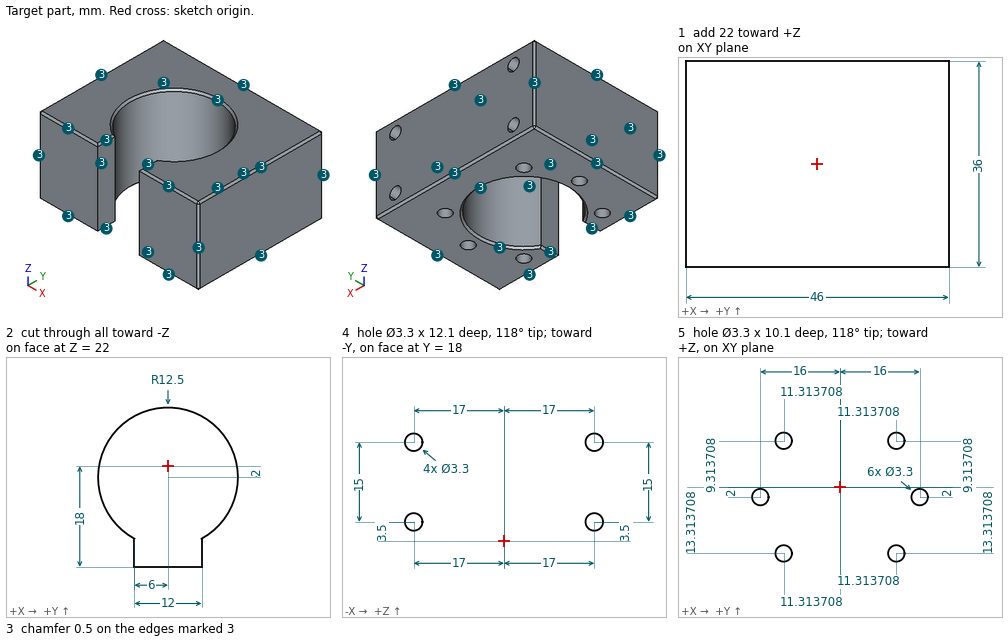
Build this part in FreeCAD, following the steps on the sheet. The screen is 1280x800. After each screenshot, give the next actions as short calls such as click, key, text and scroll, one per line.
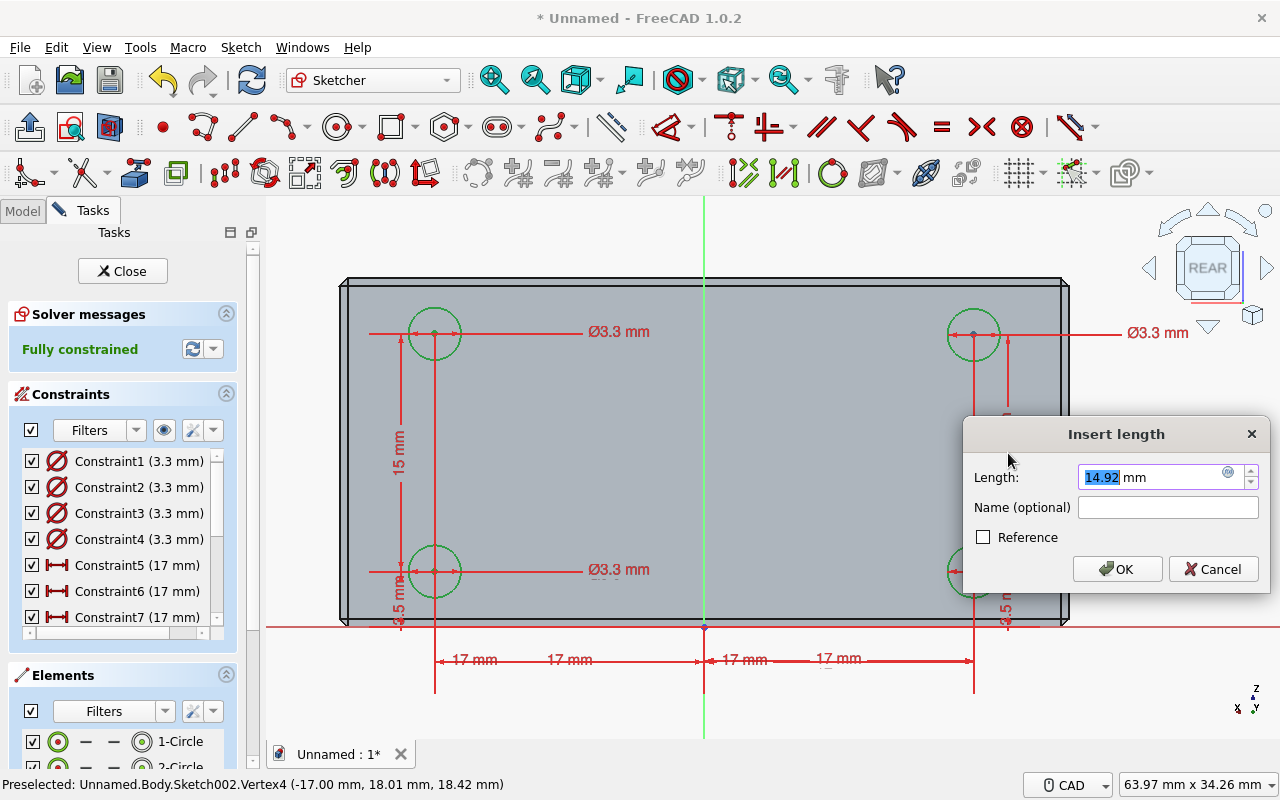
text(15)
key(Return)
key(Escape)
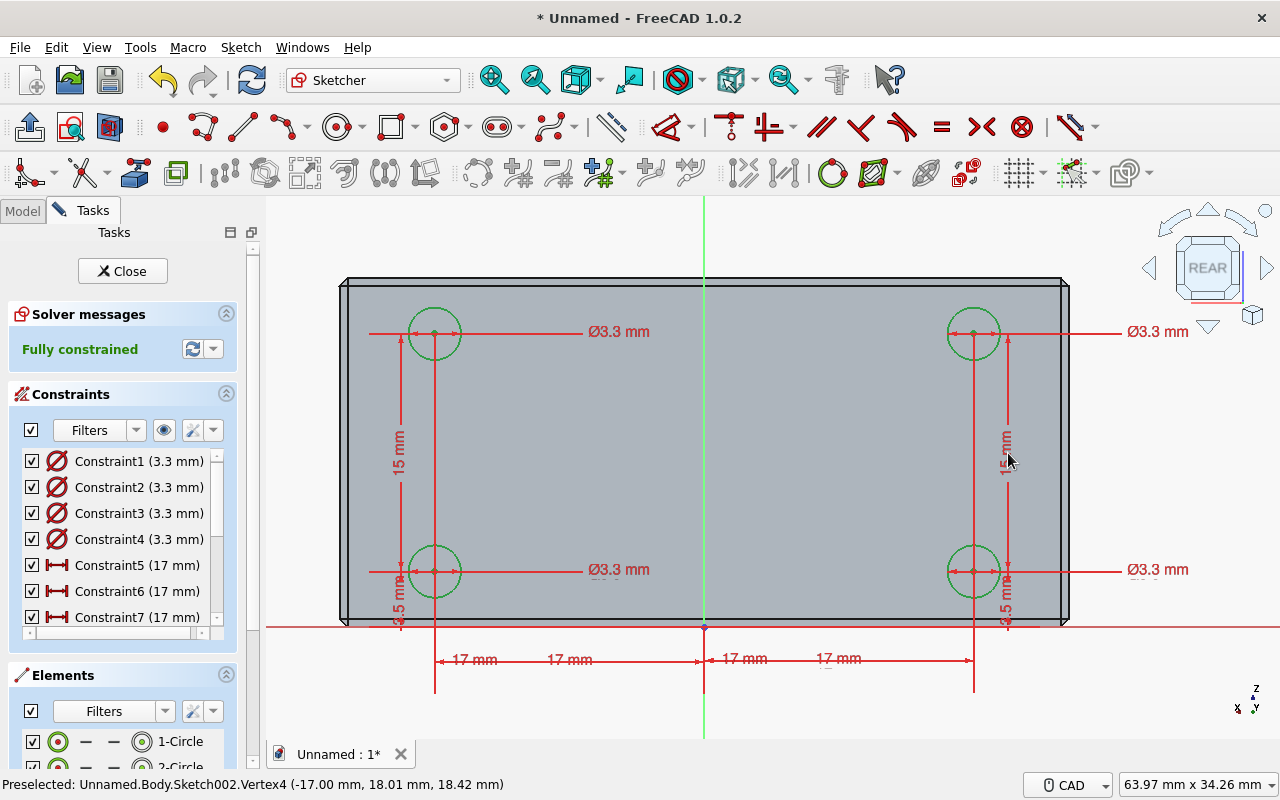
click(123, 271)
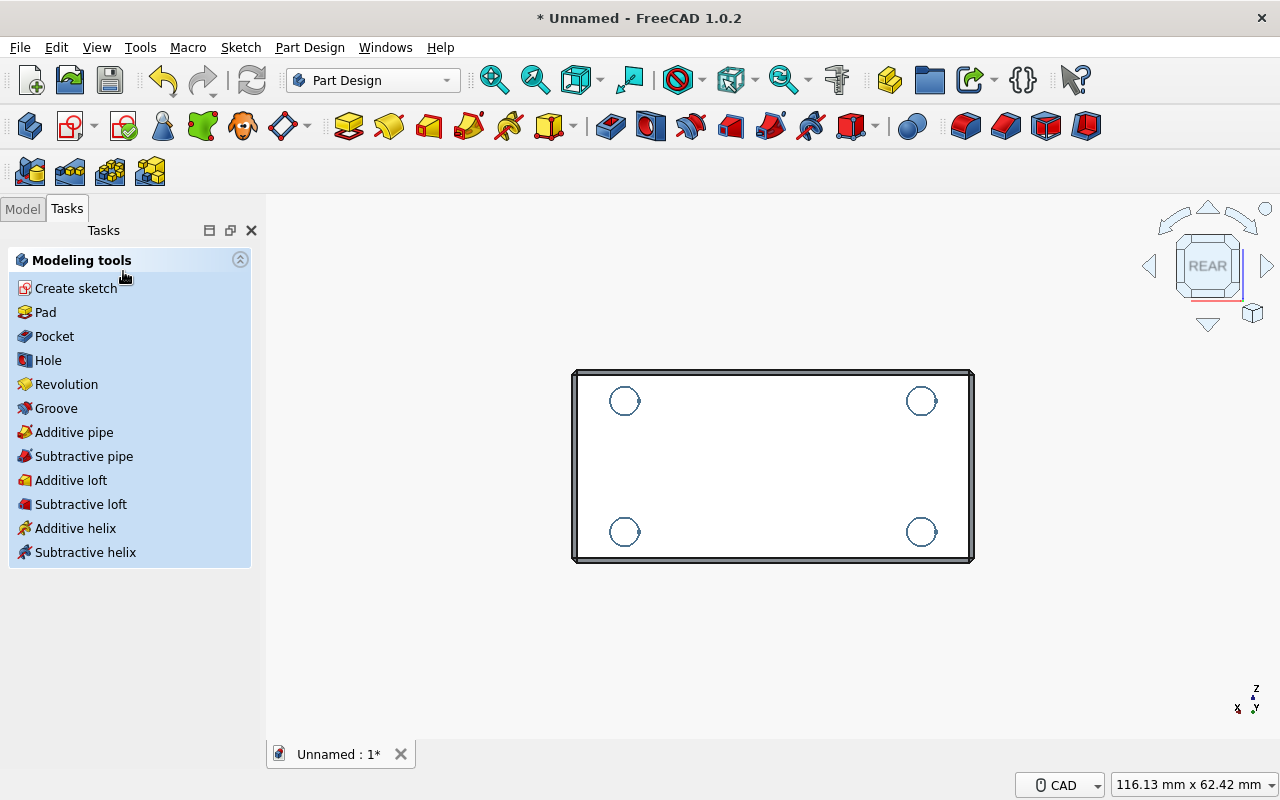
click(652, 126)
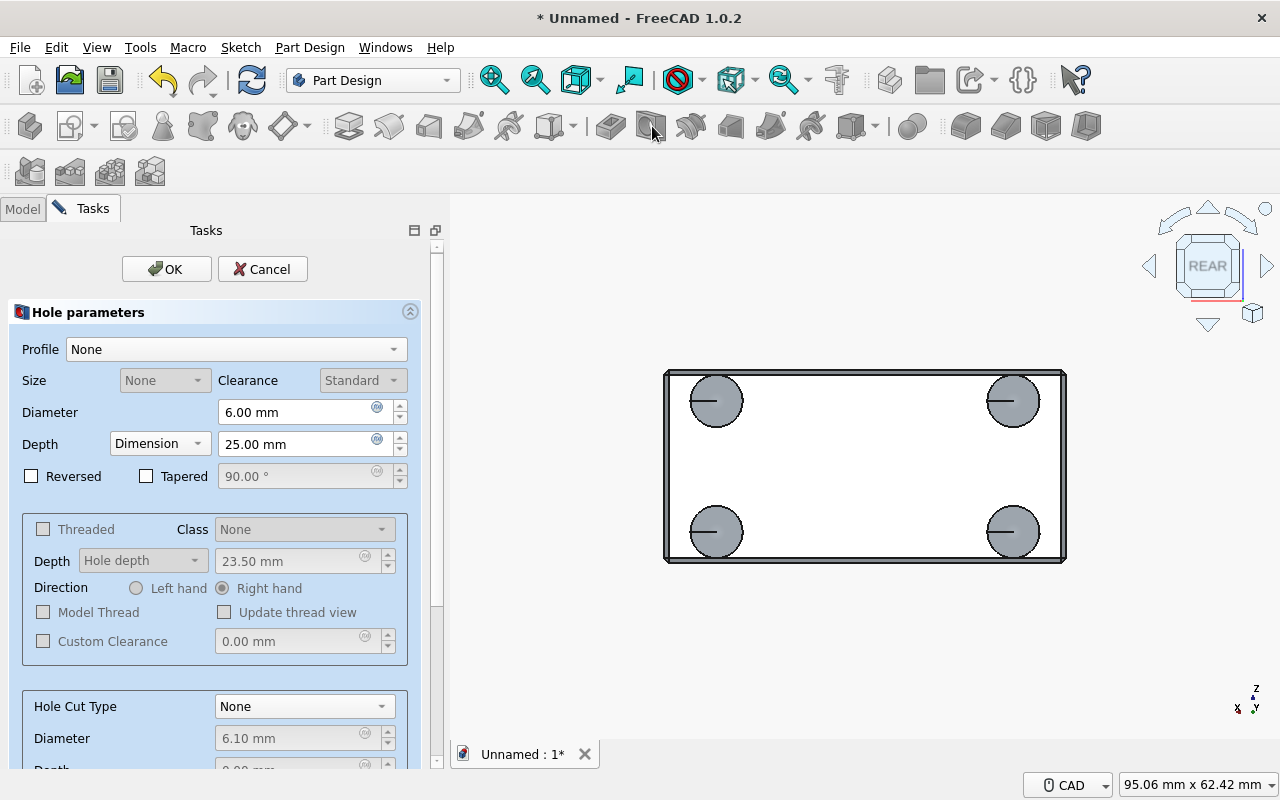
triple_click(305, 412)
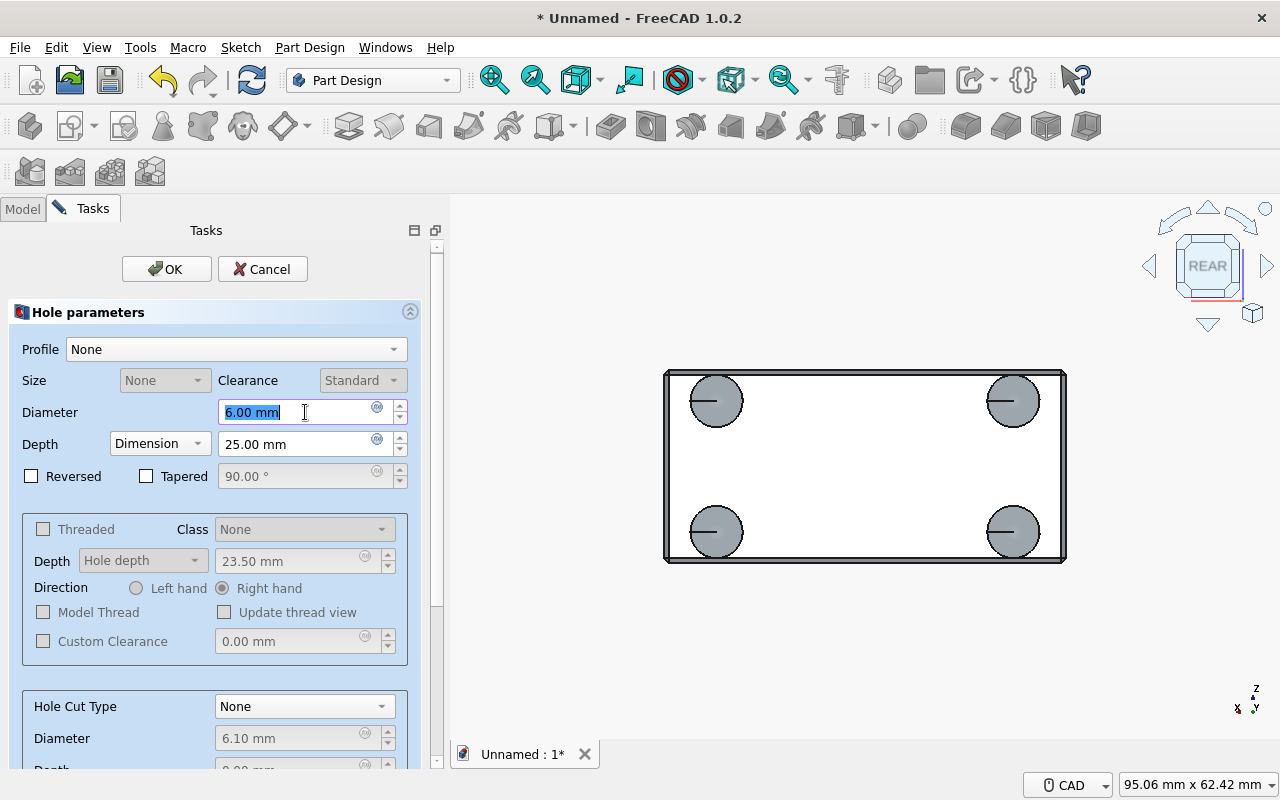
text(3.3)
key(Tab)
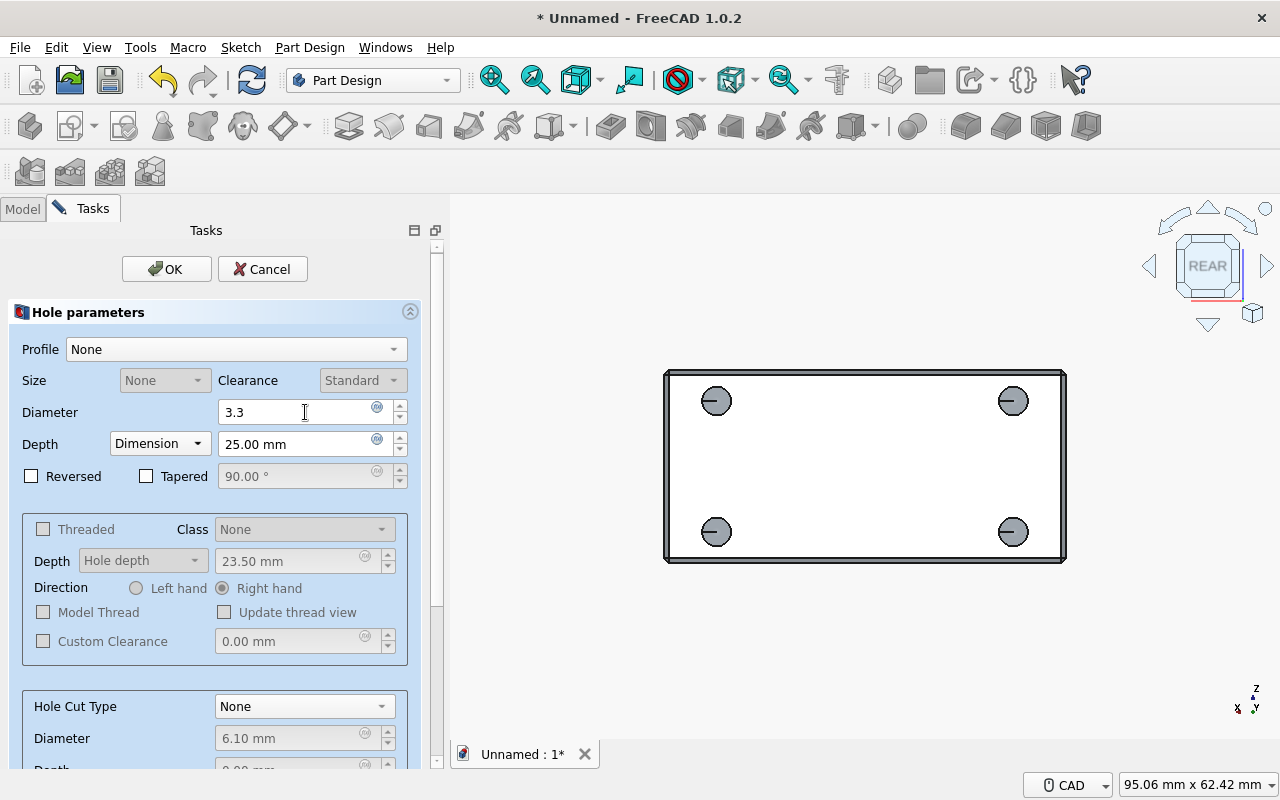
triple_click(305, 444)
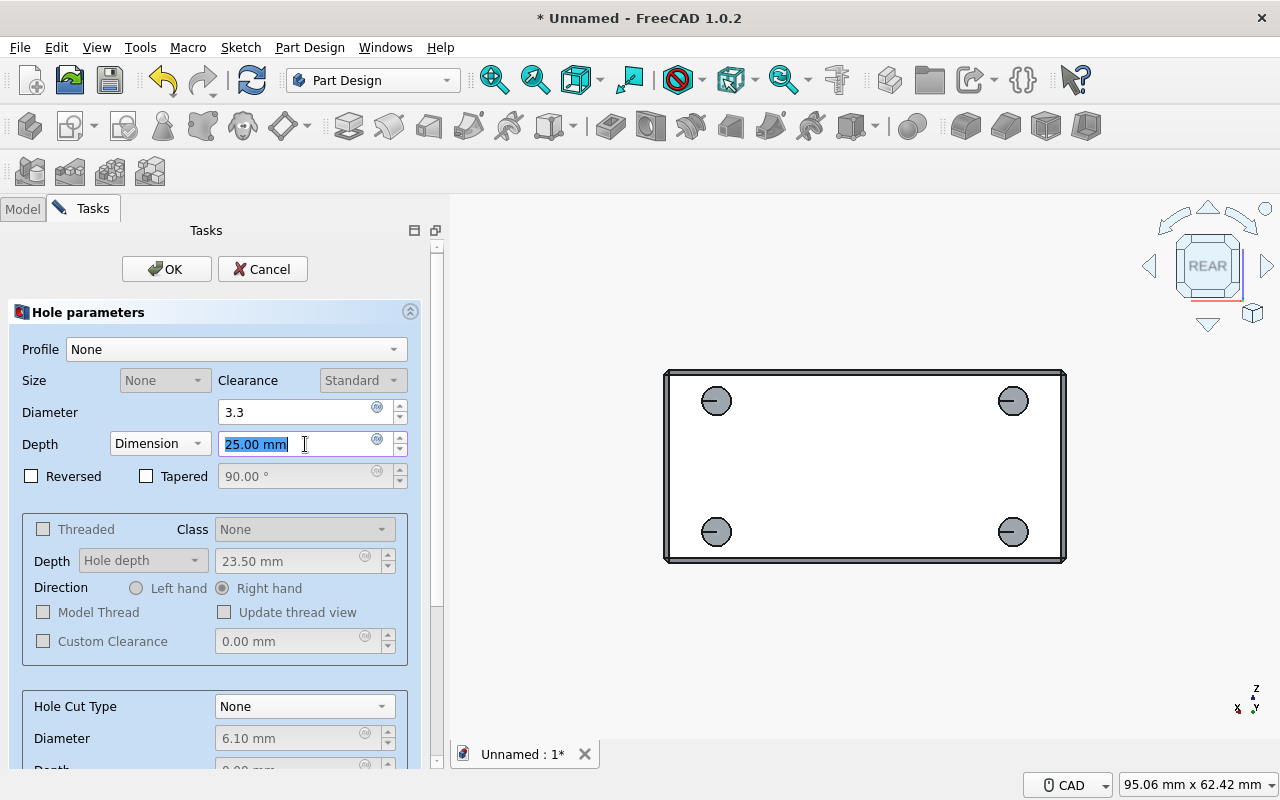
text(12.1)
key(Tab)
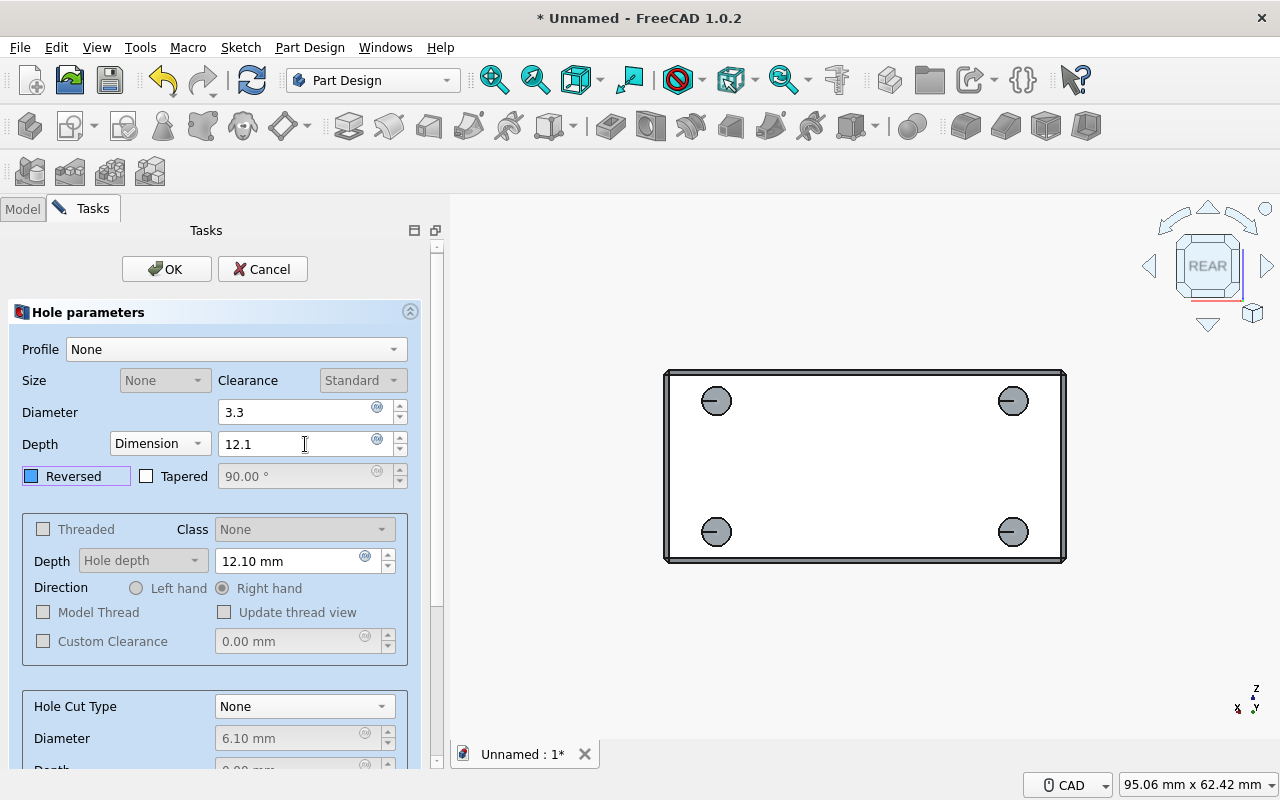
click(167, 269)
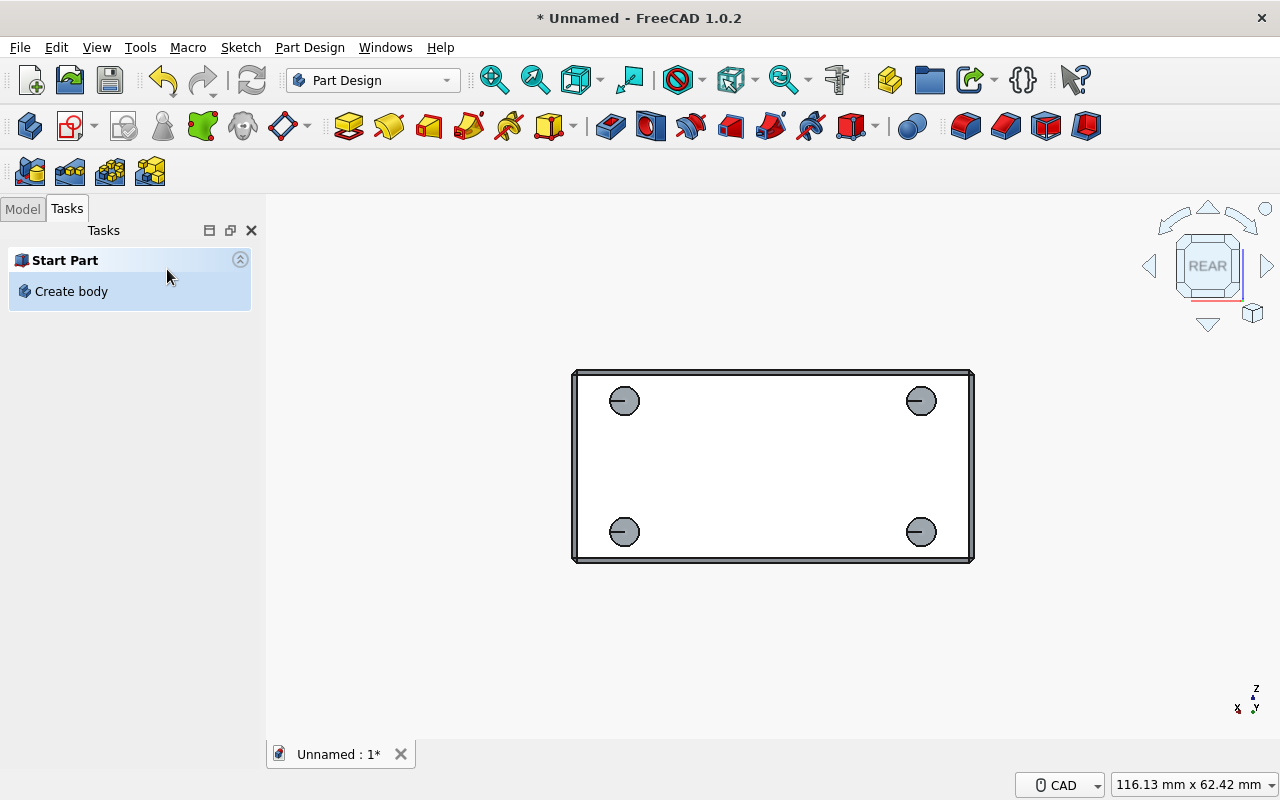
click(496, 80)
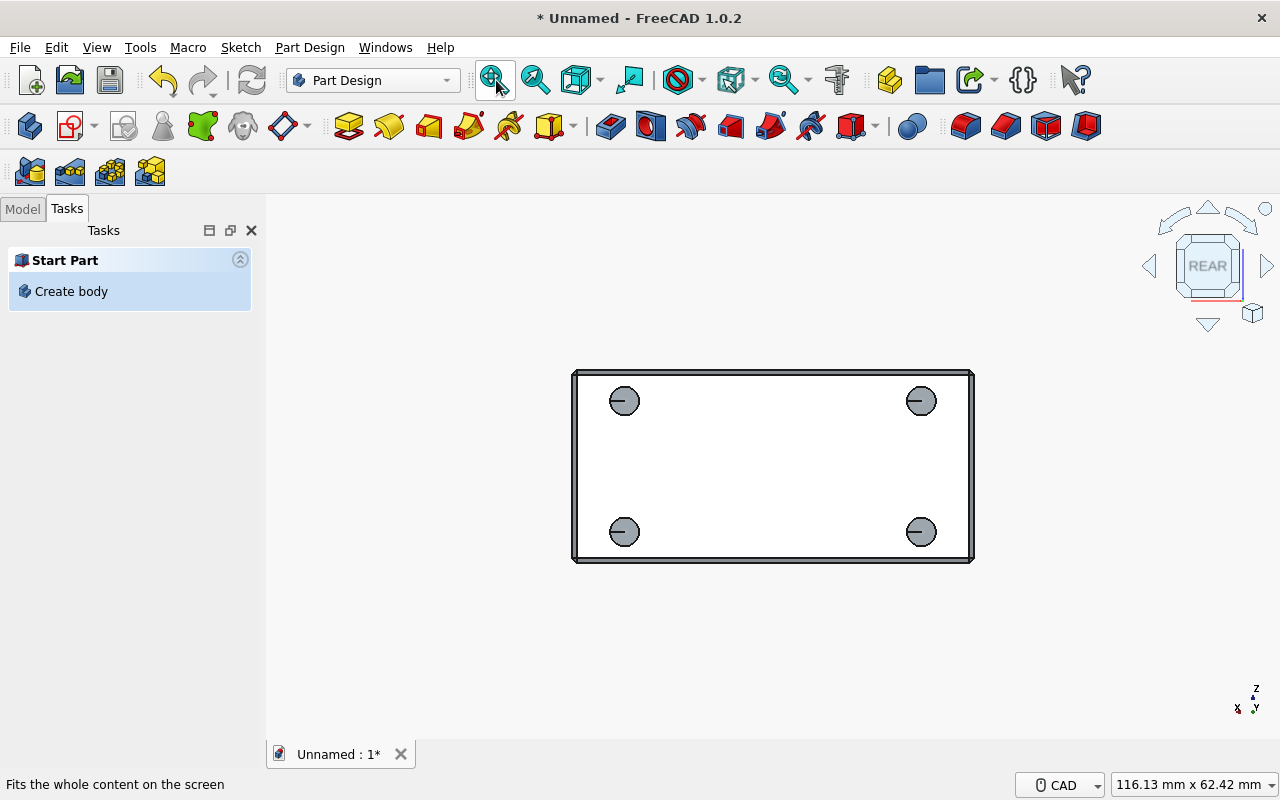
click(70, 126)